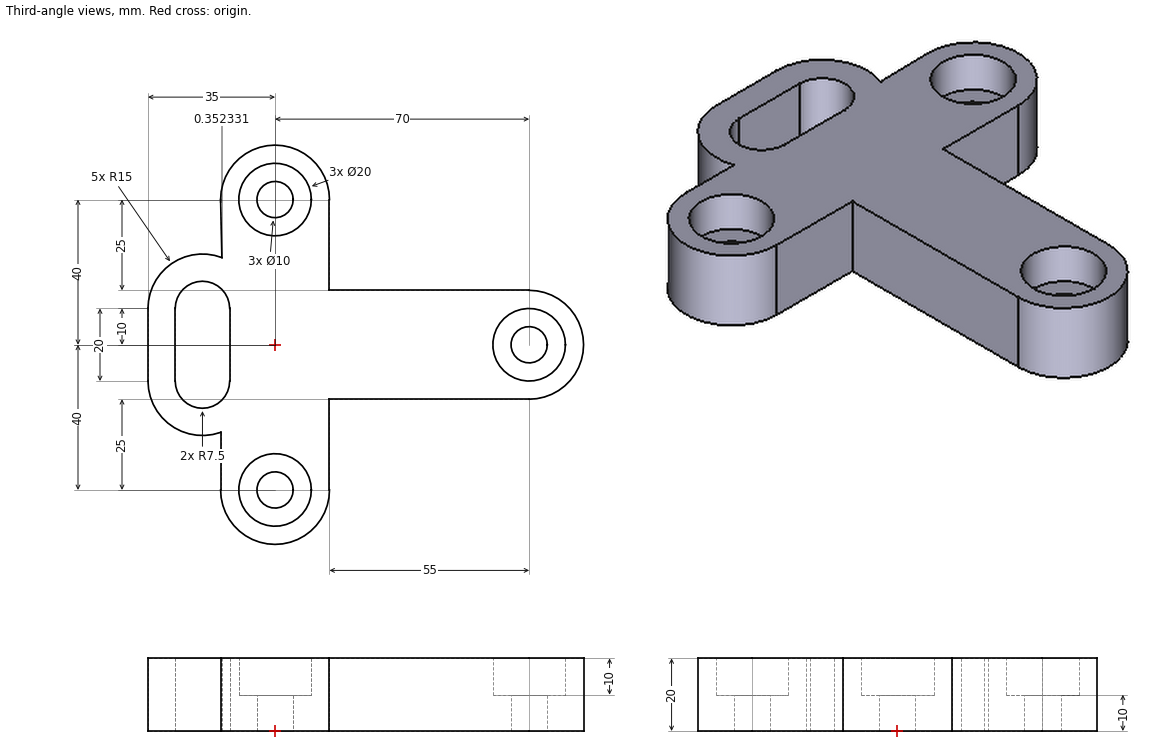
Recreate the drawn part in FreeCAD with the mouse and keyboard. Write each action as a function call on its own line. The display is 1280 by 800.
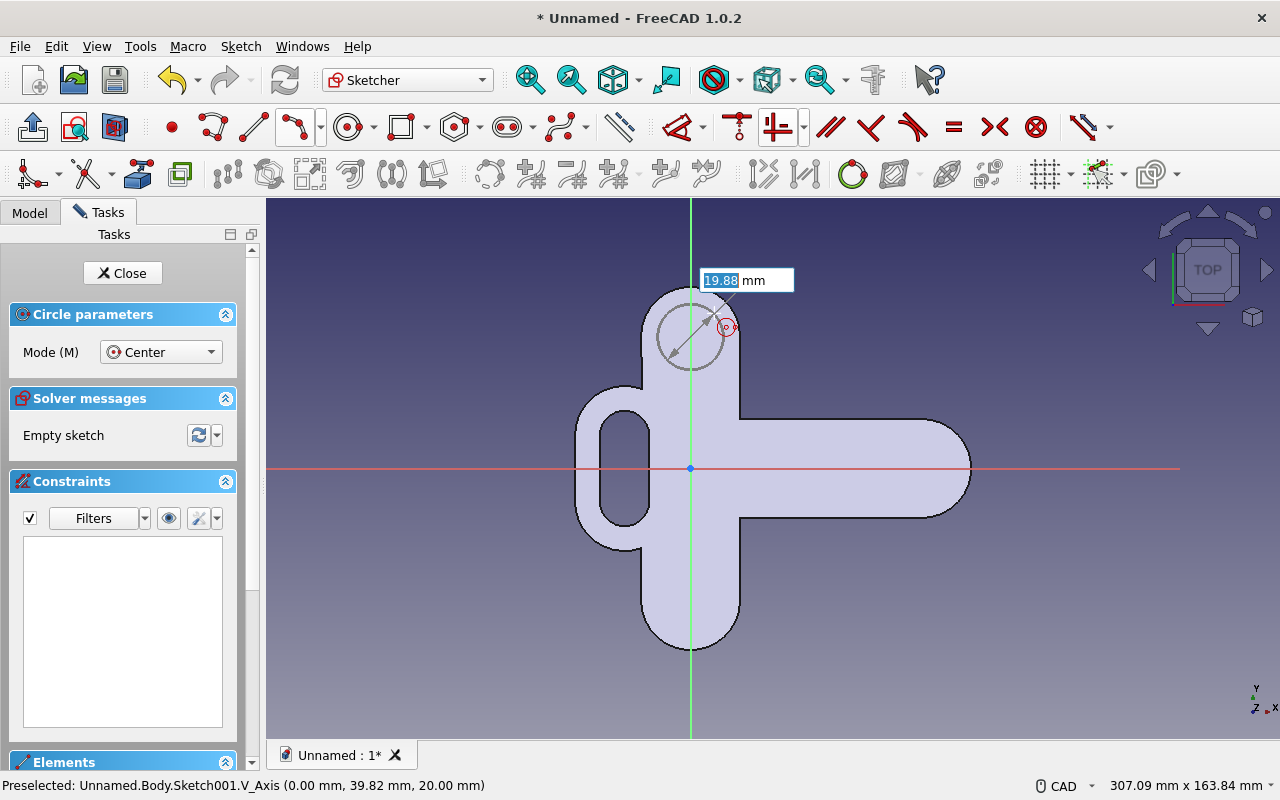
text(20)
key(Return)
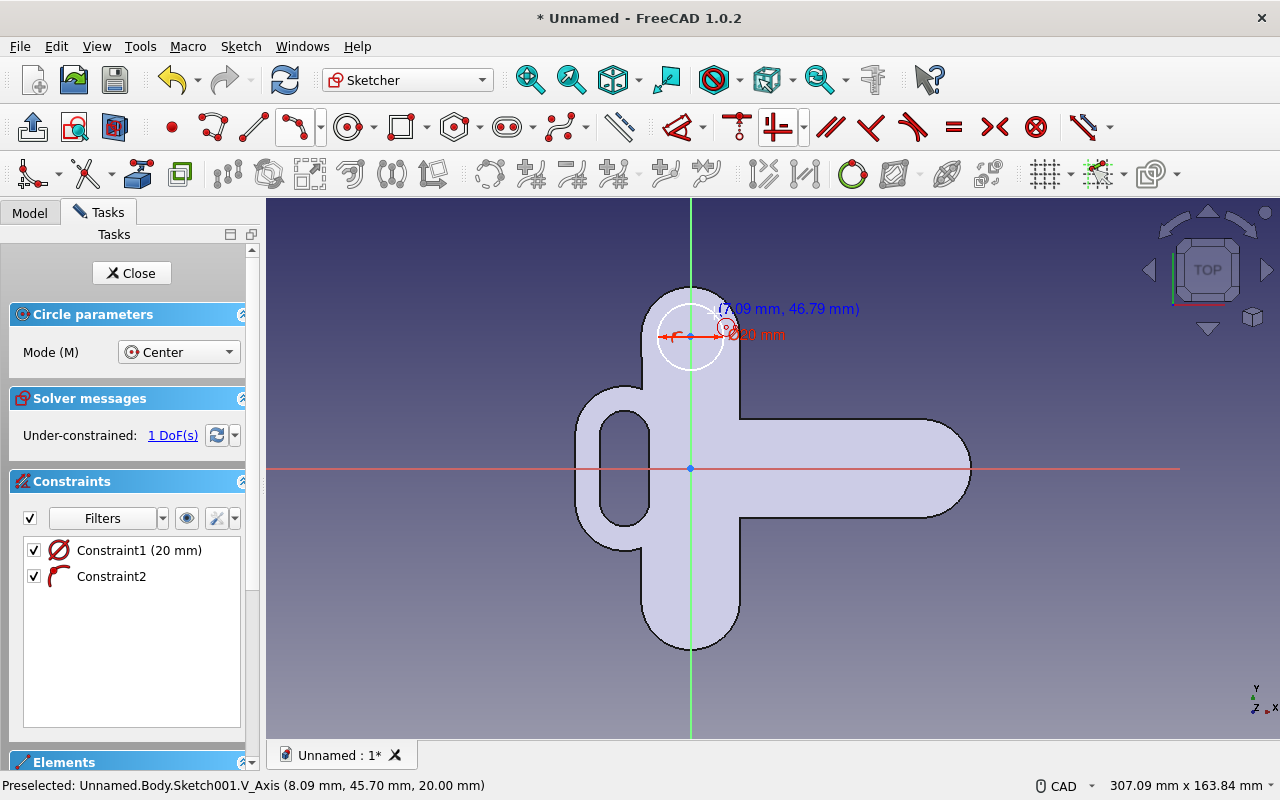
click(691, 601)
move(714, 577)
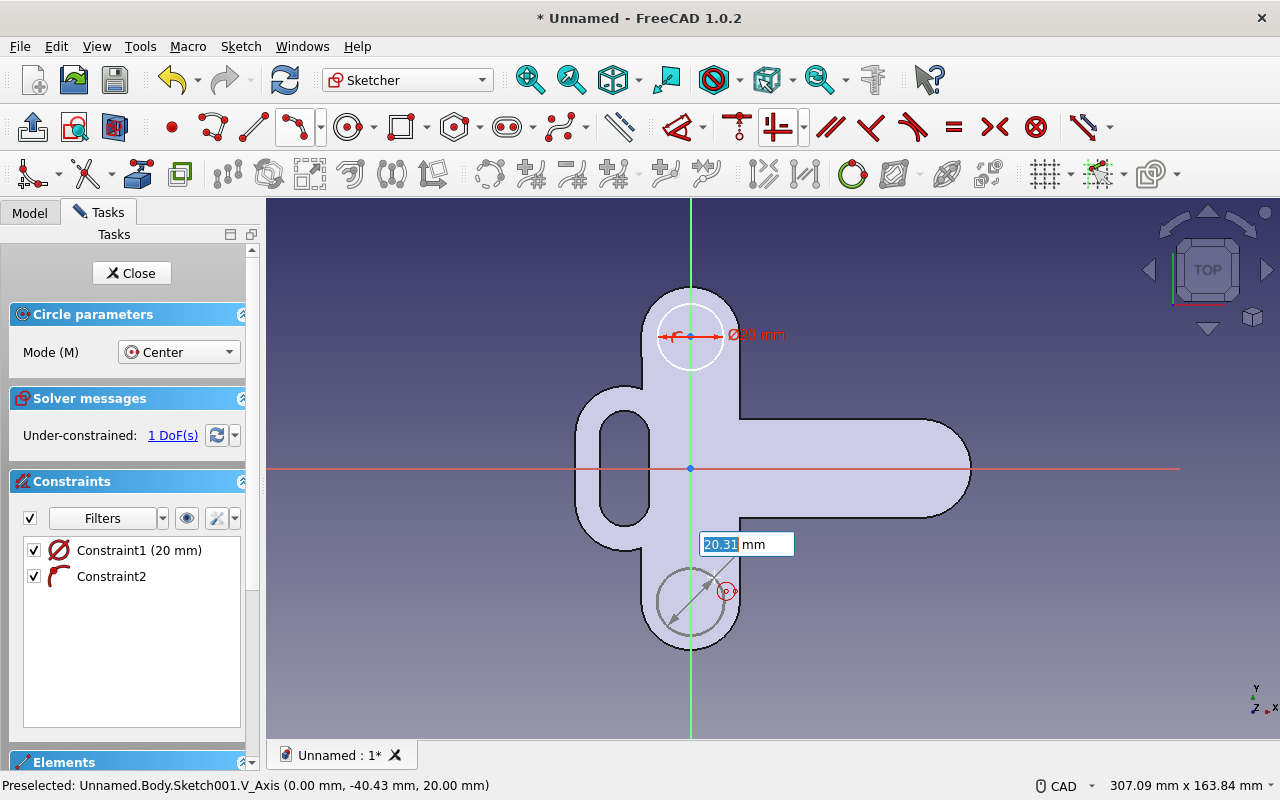
text(20)
key(Return)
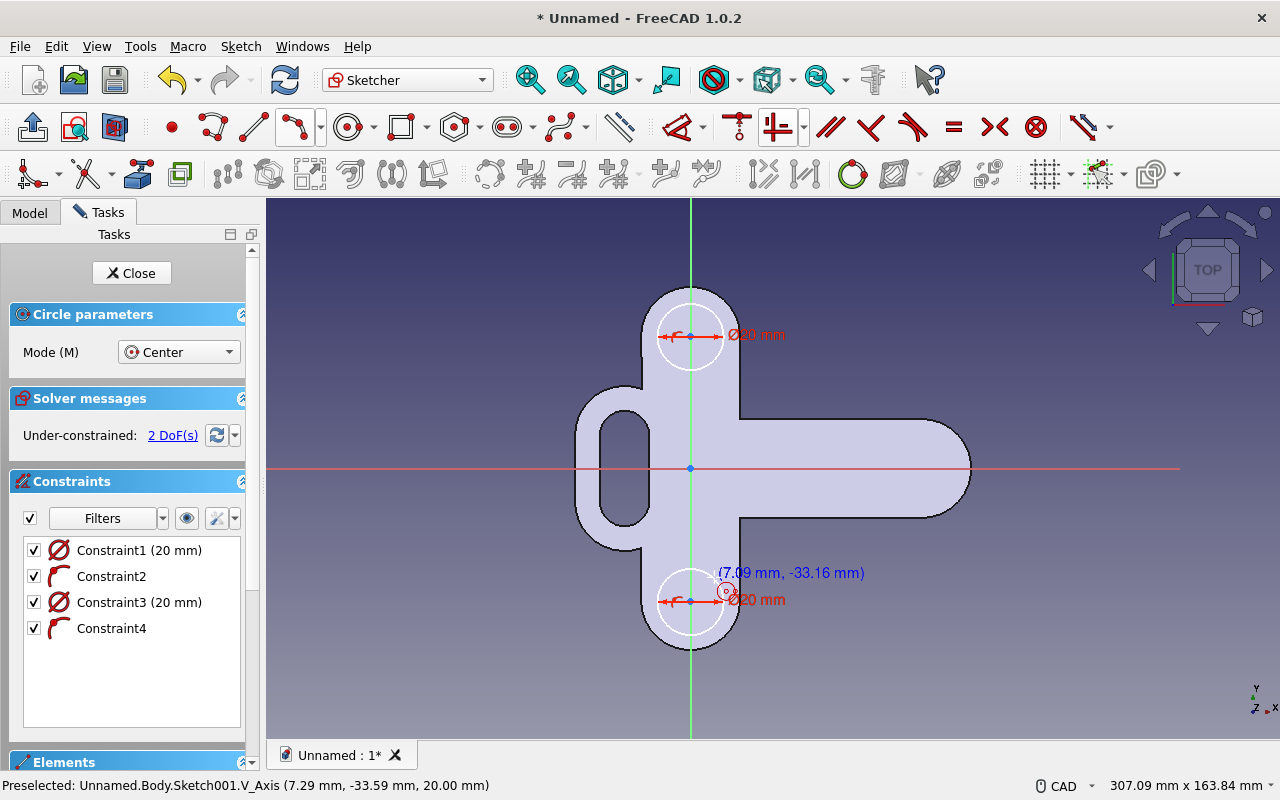
click(922, 468)
move(945, 445)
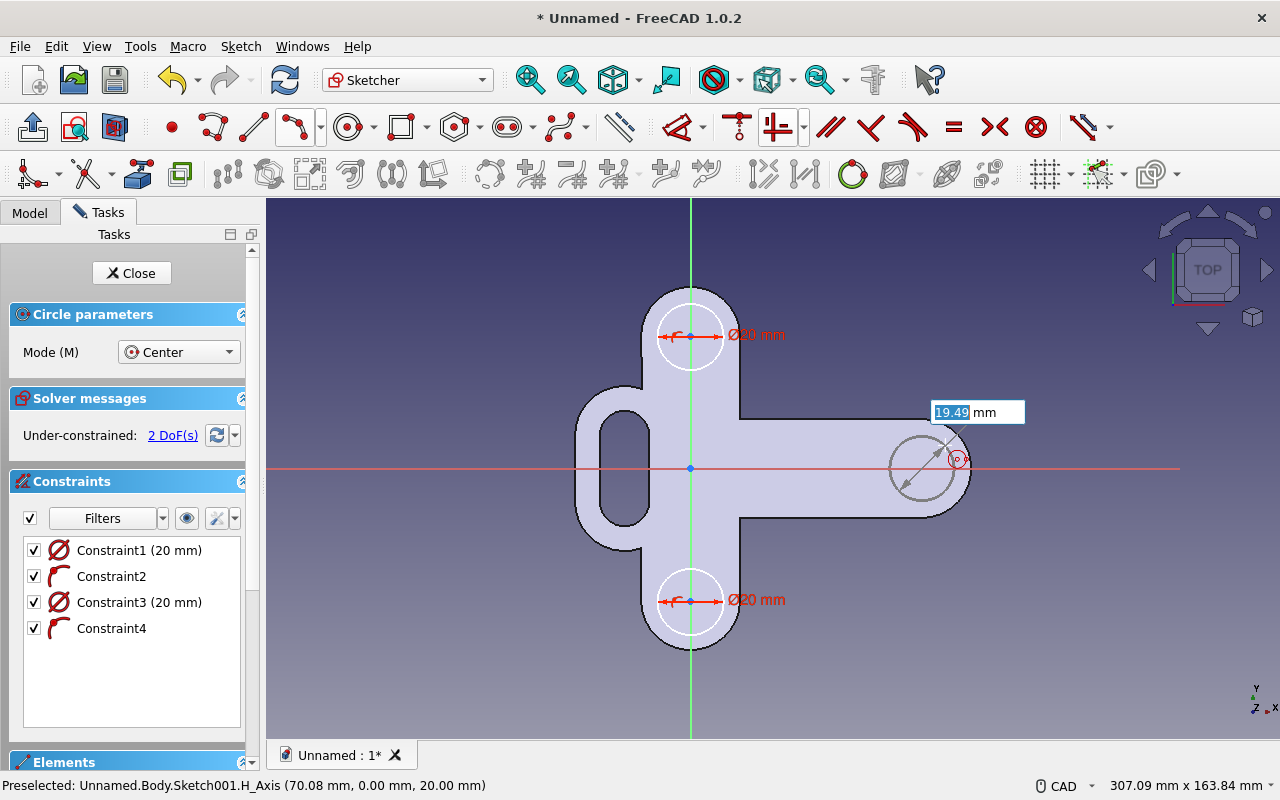
text(20)
key(Return)
key(Escape)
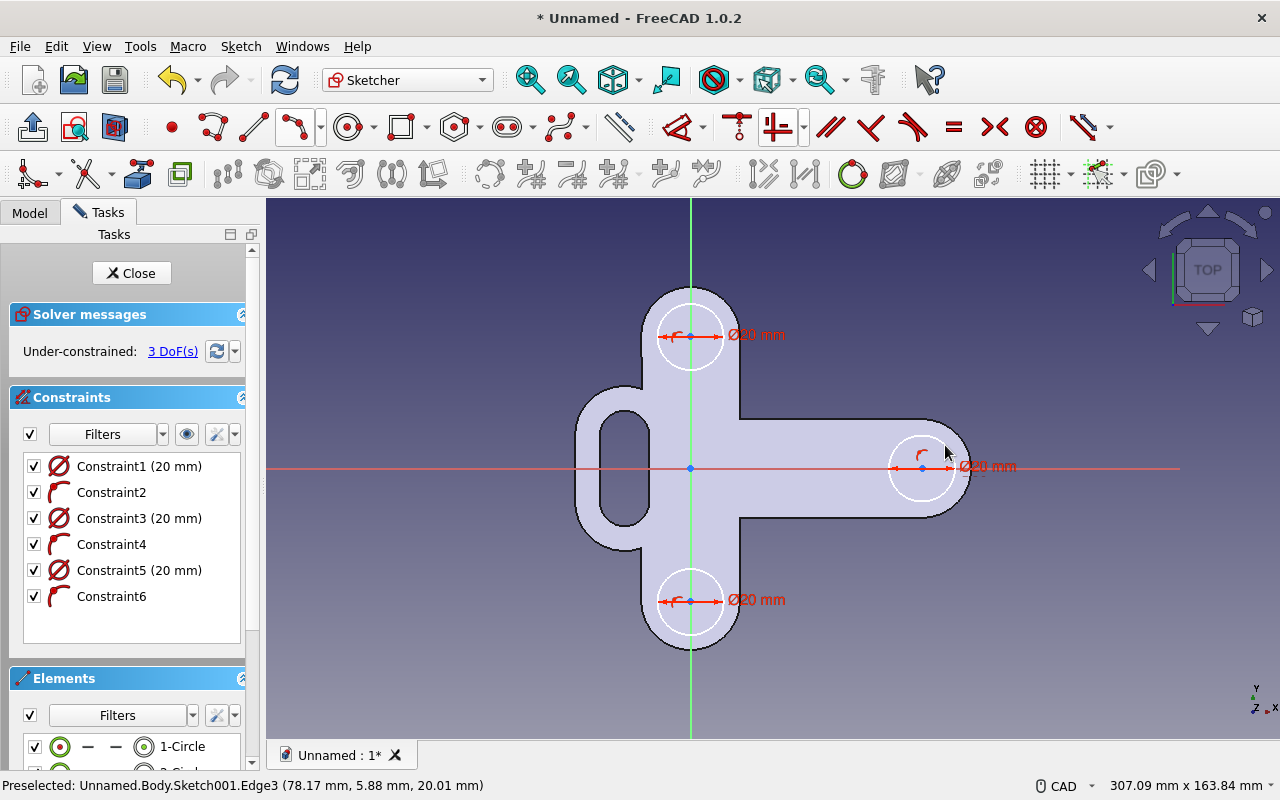
click(691, 337)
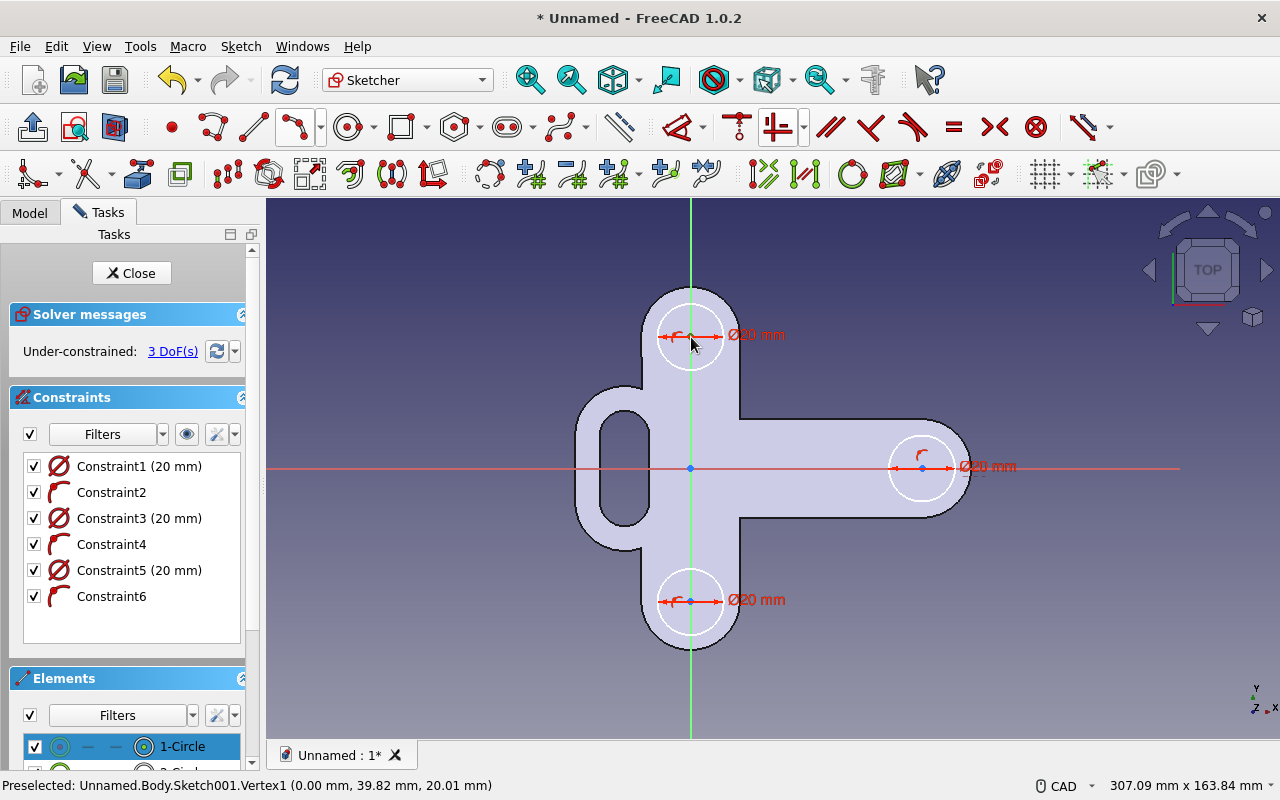
click(702, 128)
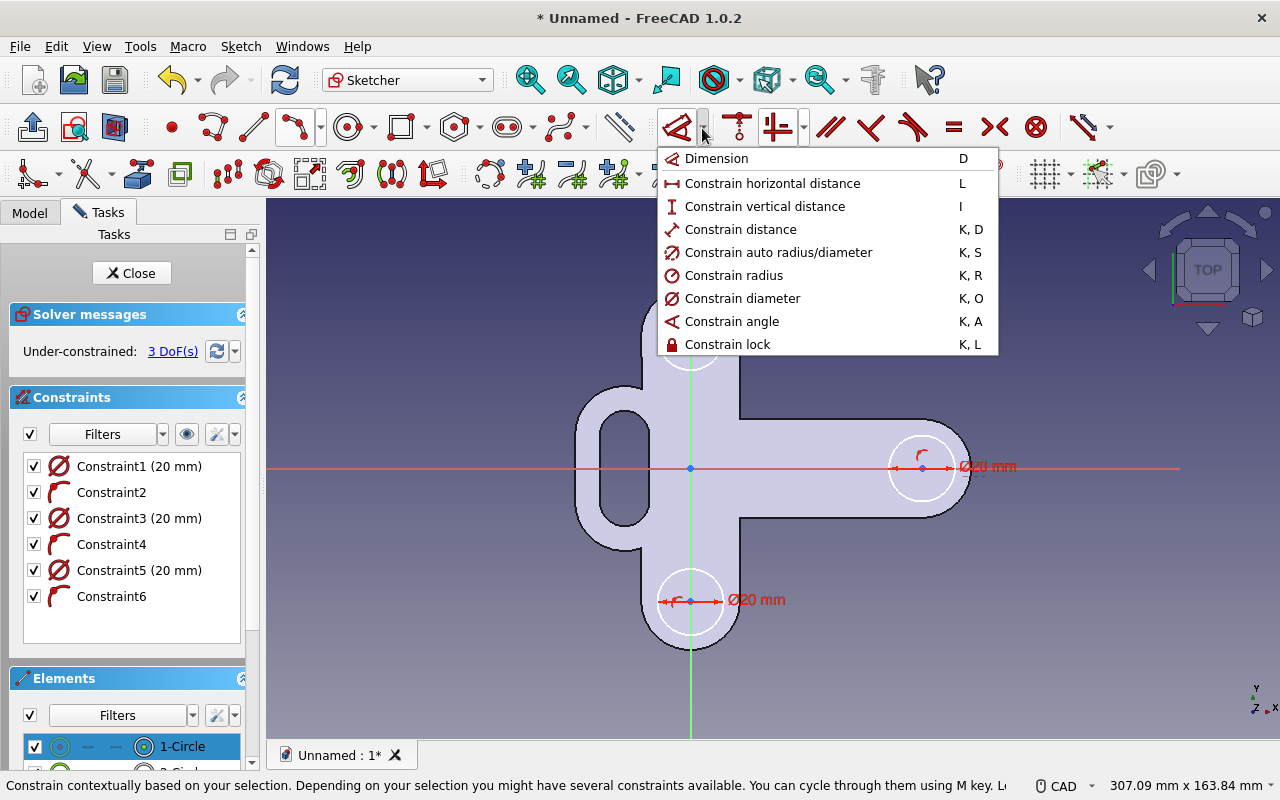
click(828, 206)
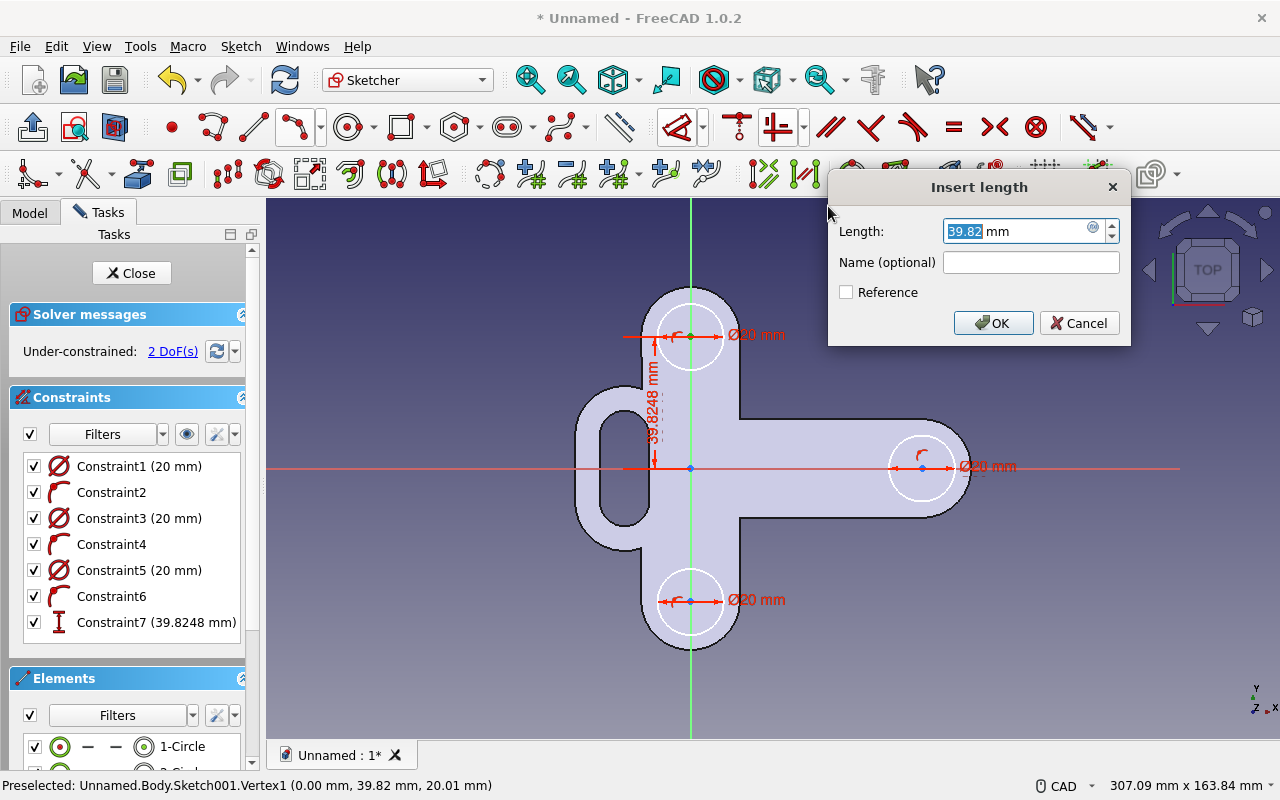
text(40)
key(Return)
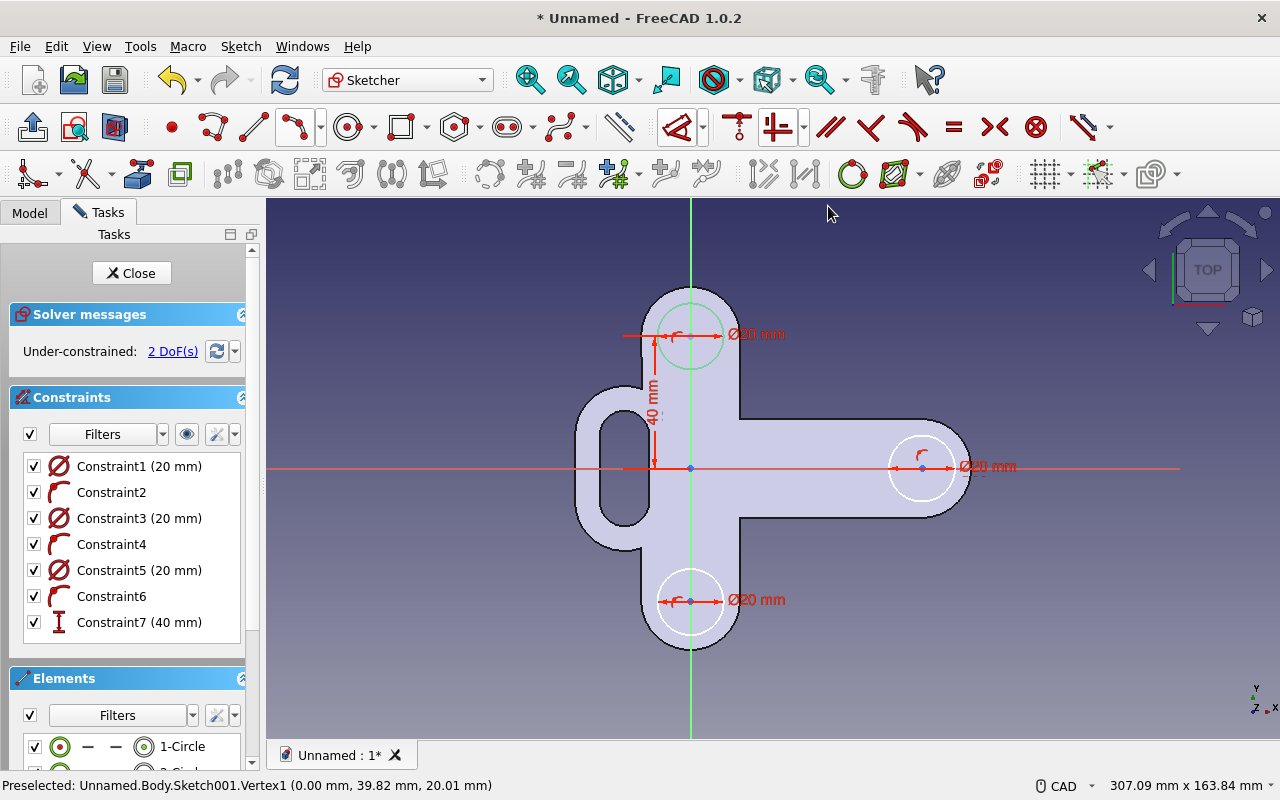
click(691, 602)